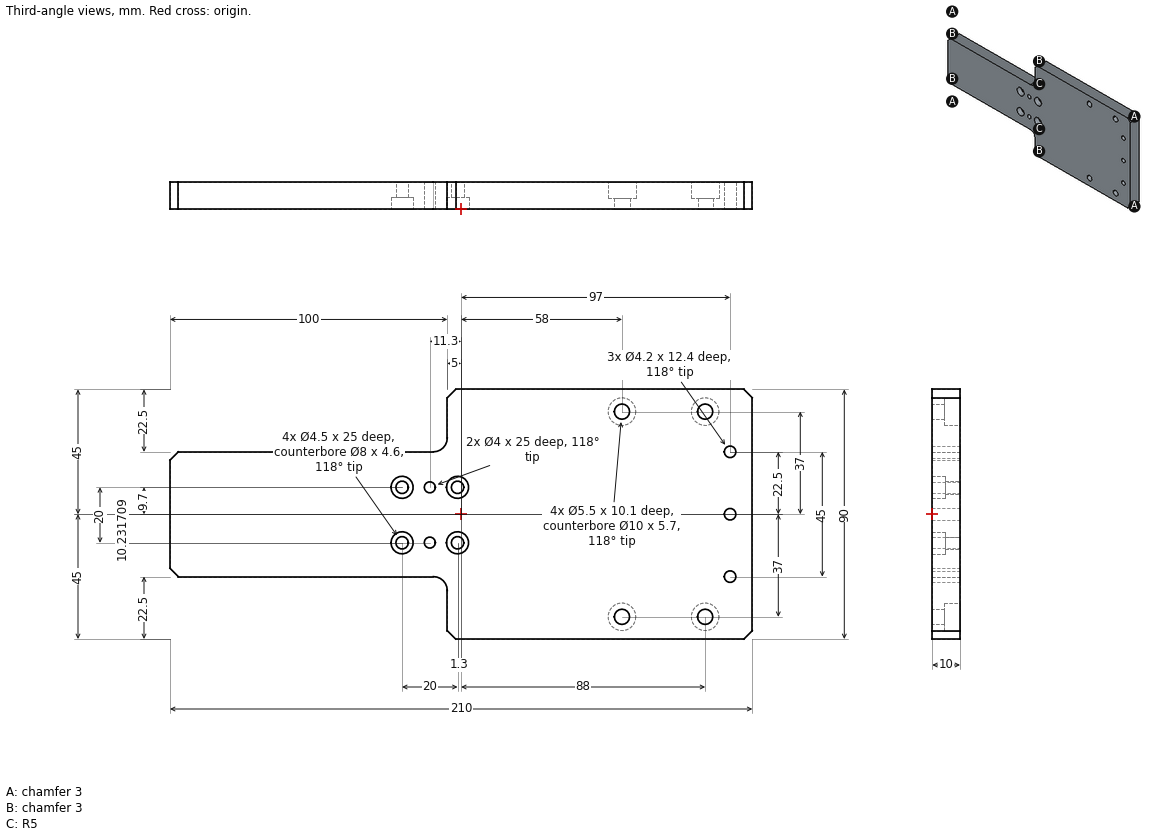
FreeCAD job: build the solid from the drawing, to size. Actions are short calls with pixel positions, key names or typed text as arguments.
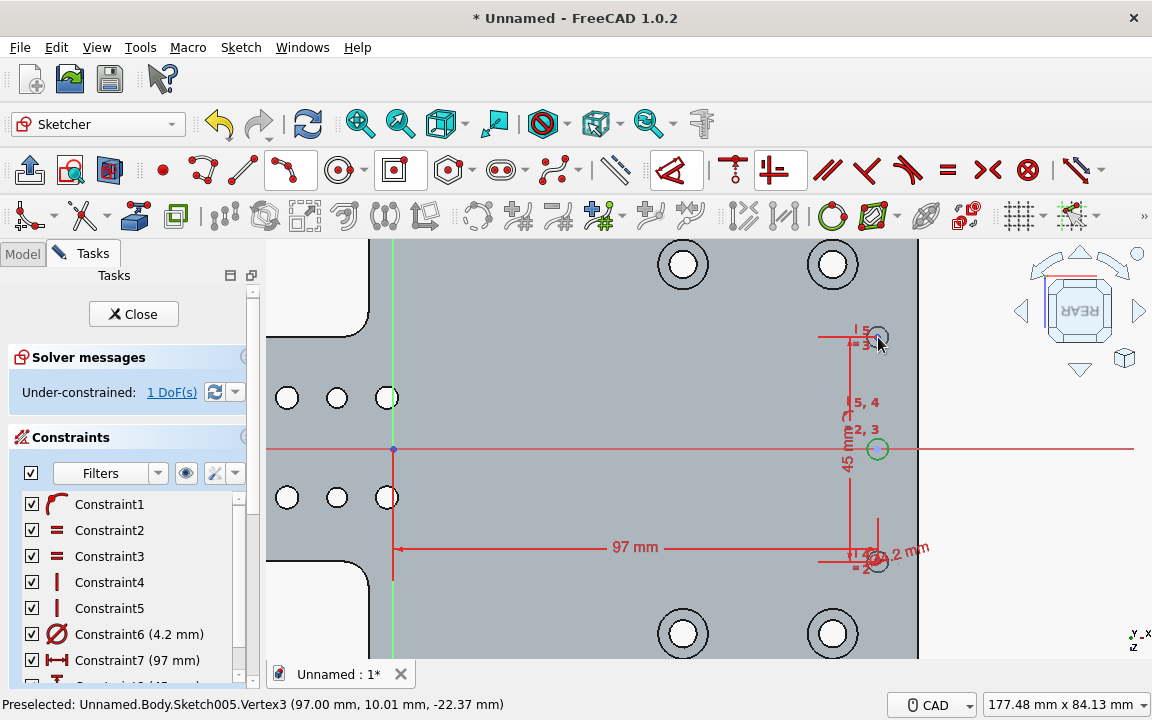
click(878, 562)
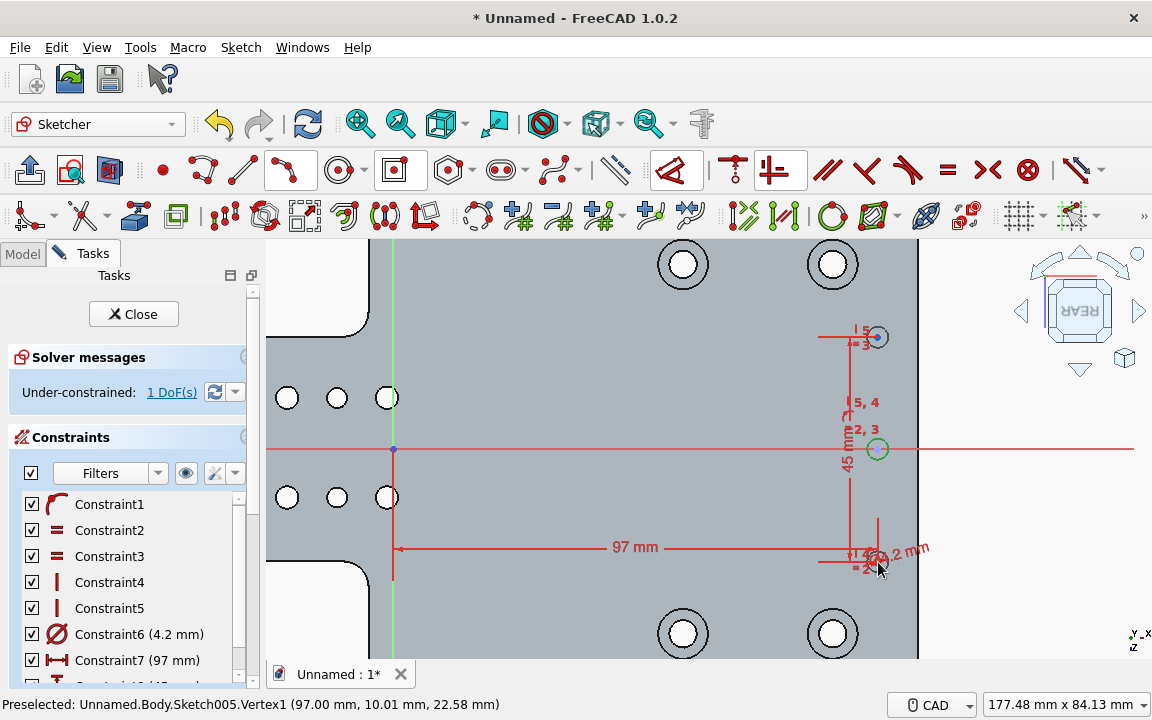
key(i)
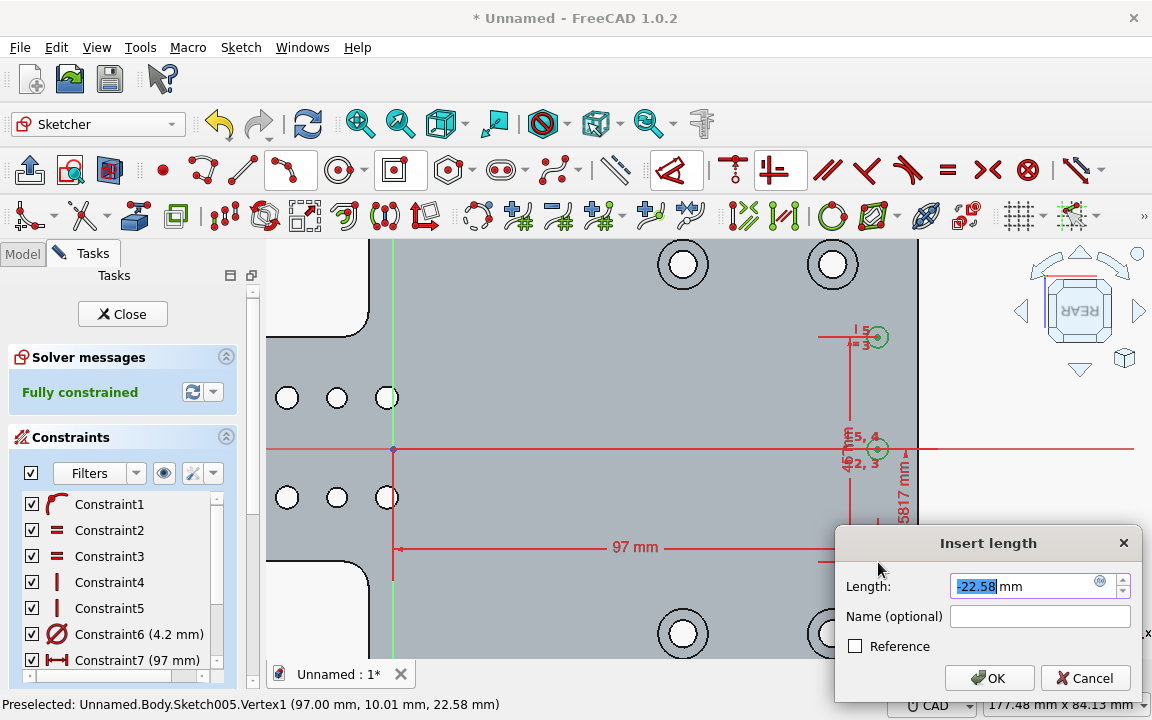
text(-22.5)
key(Return)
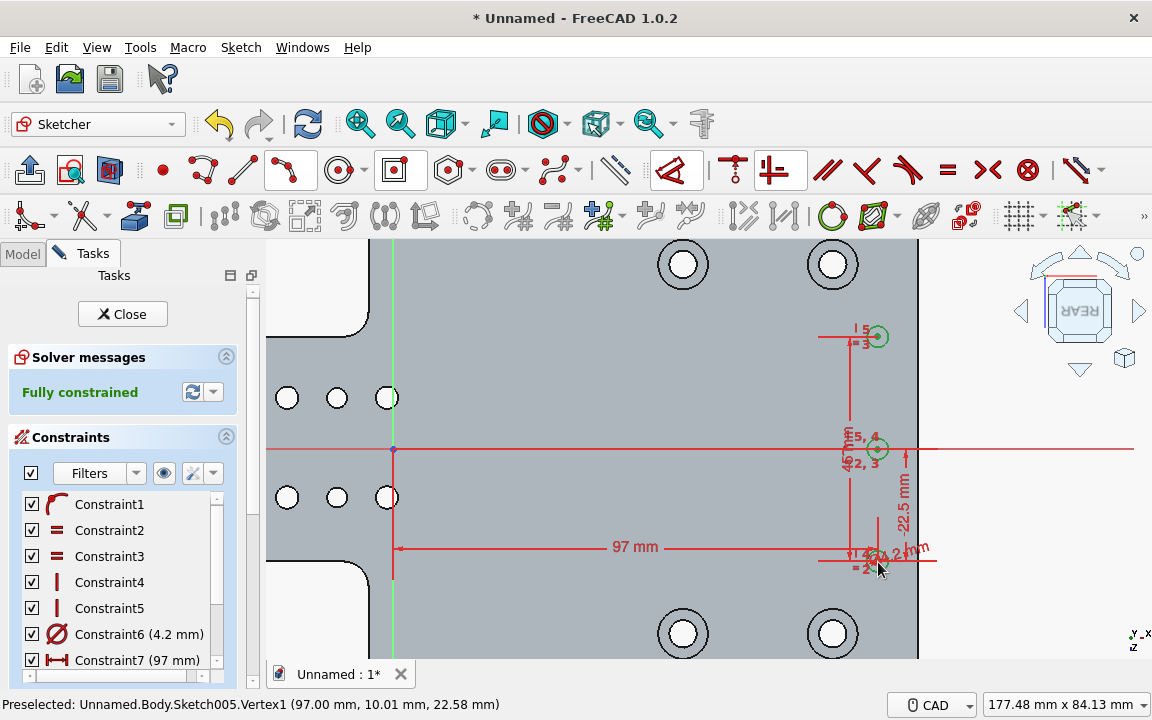
click(123, 314)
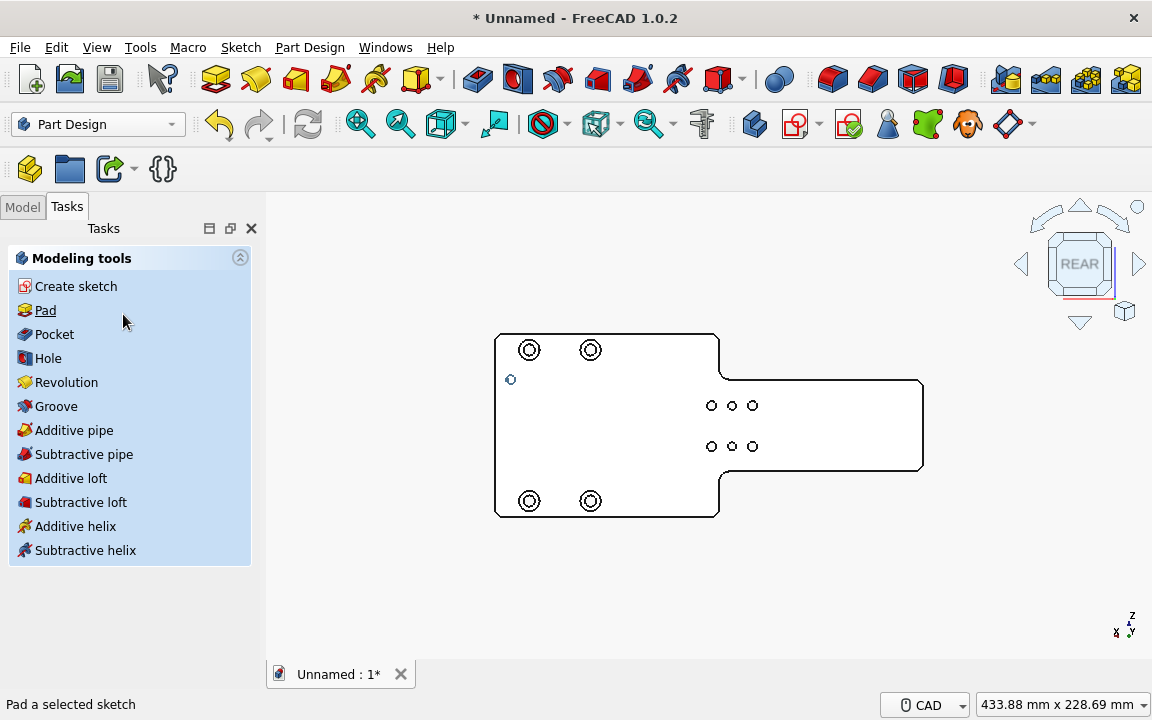
click(518, 80)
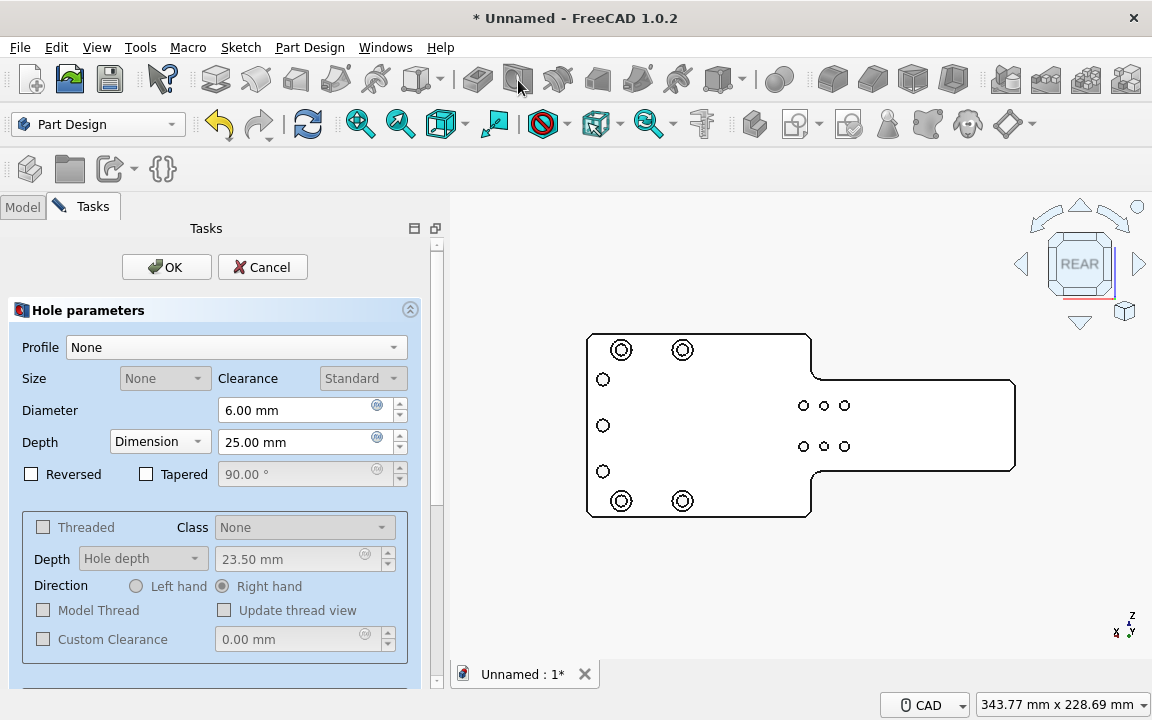
triple_click(305, 410)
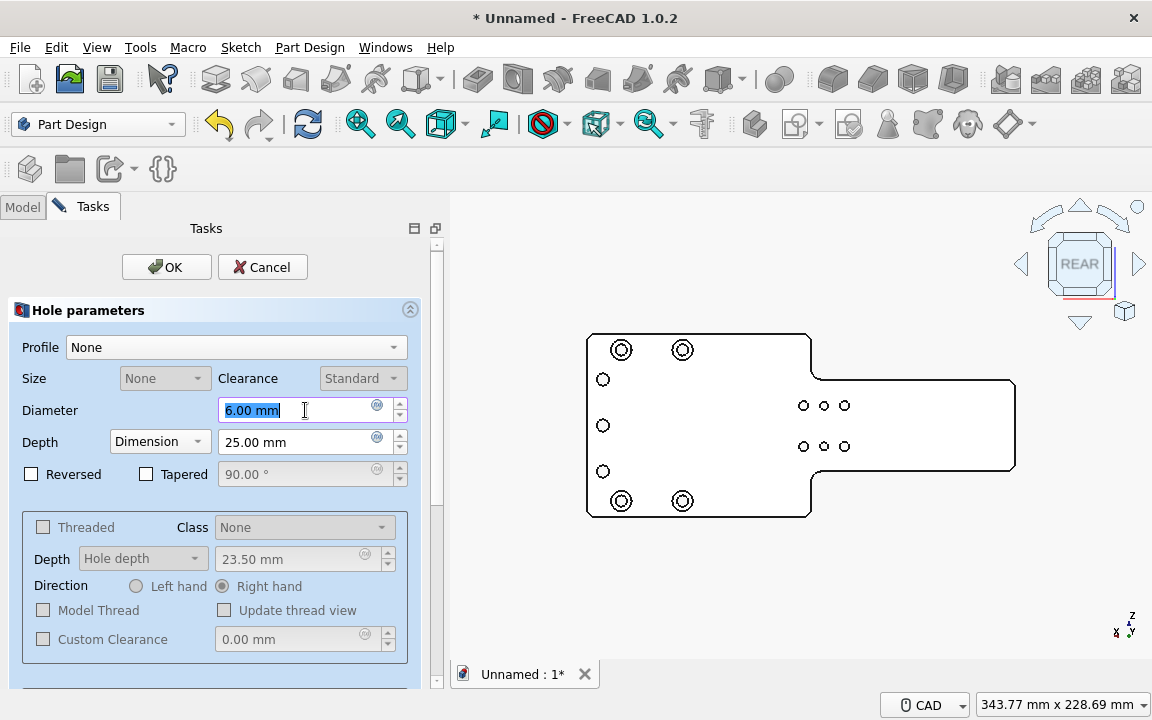
text(4.2)
key(Tab)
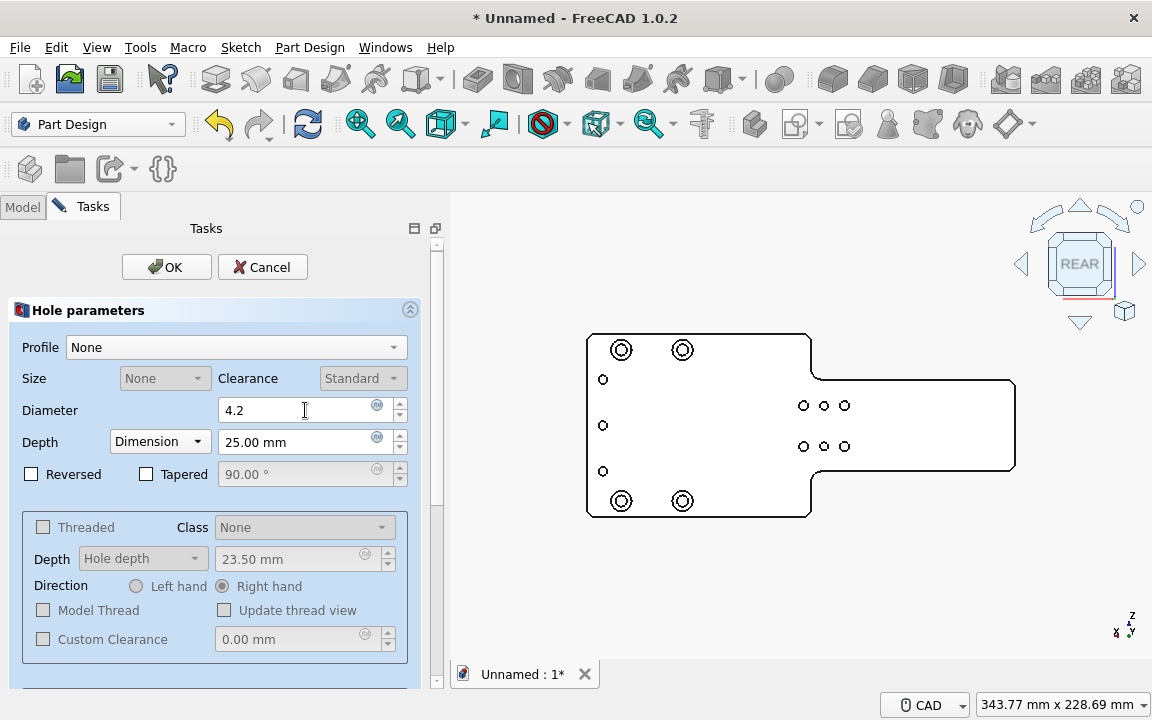
triple_click(305, 442)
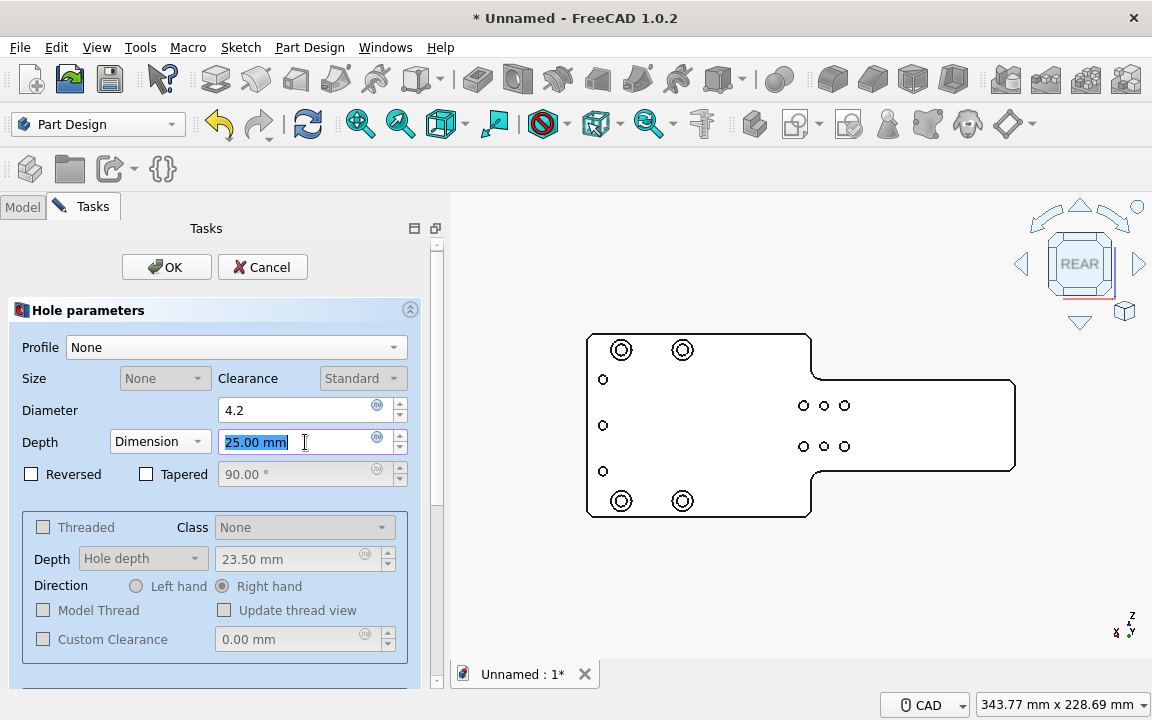
text(12.4)
key(Tab)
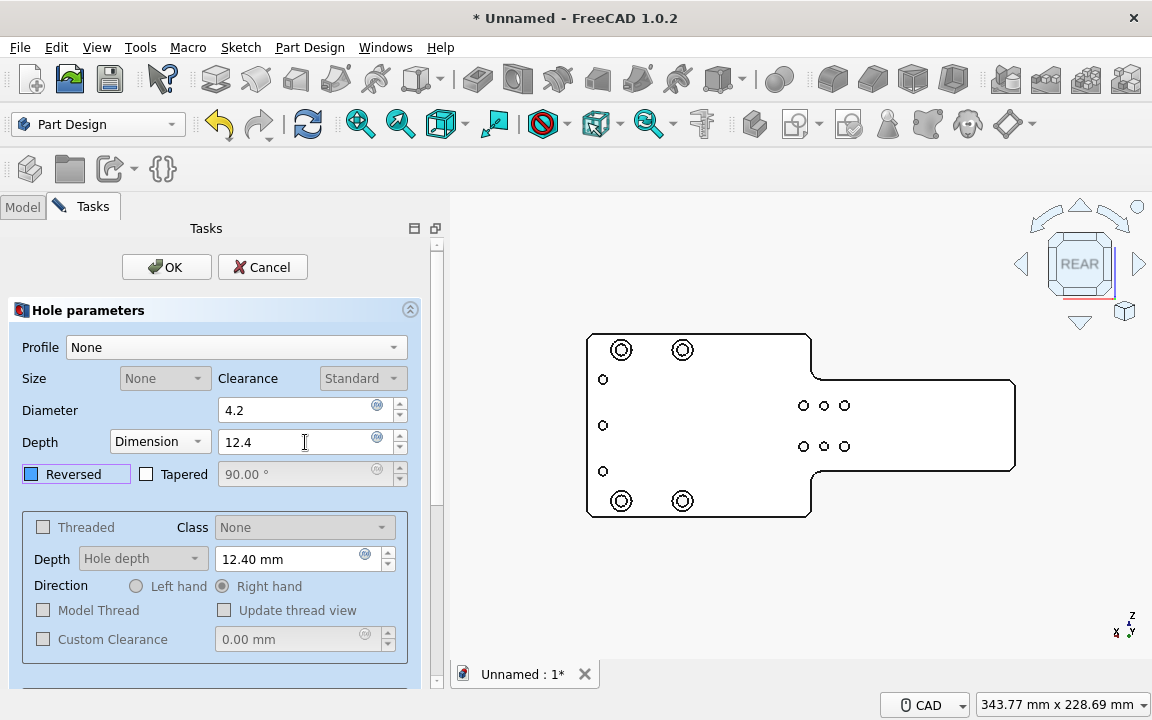
click(167, 267)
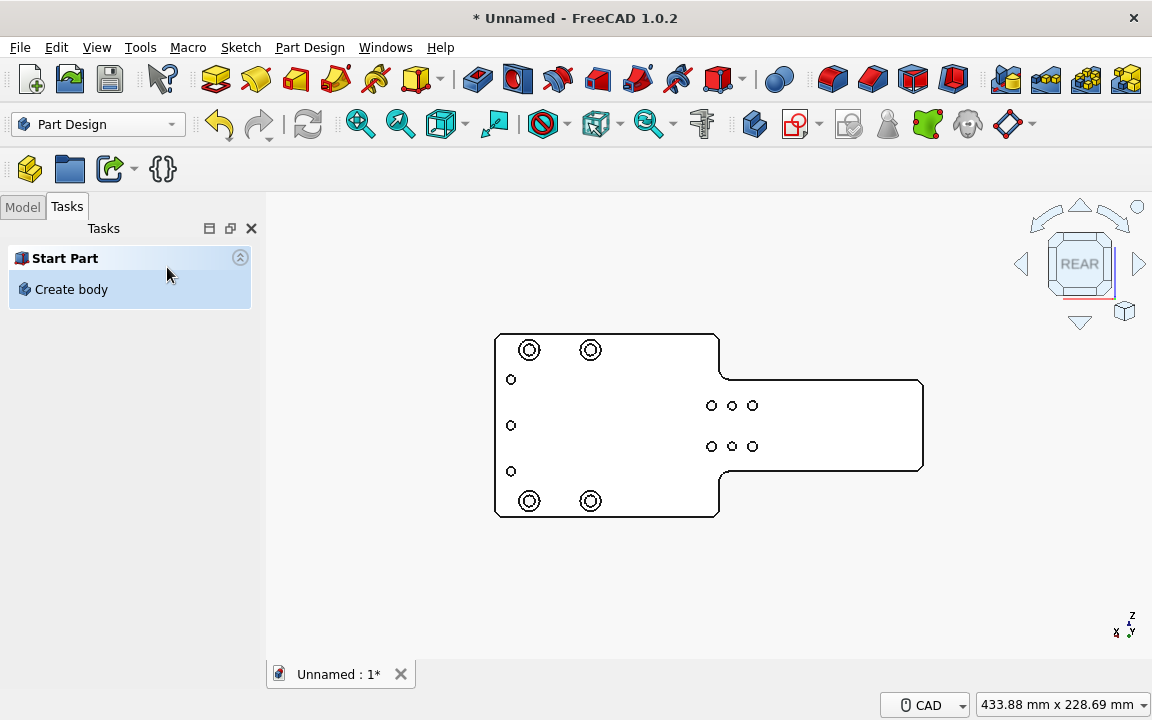
key(0)